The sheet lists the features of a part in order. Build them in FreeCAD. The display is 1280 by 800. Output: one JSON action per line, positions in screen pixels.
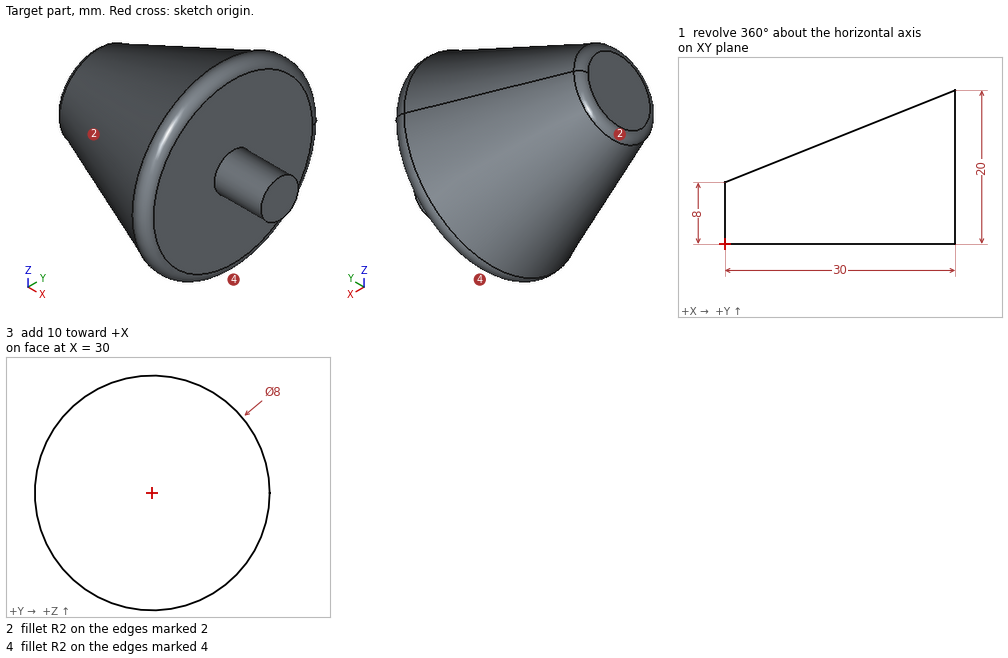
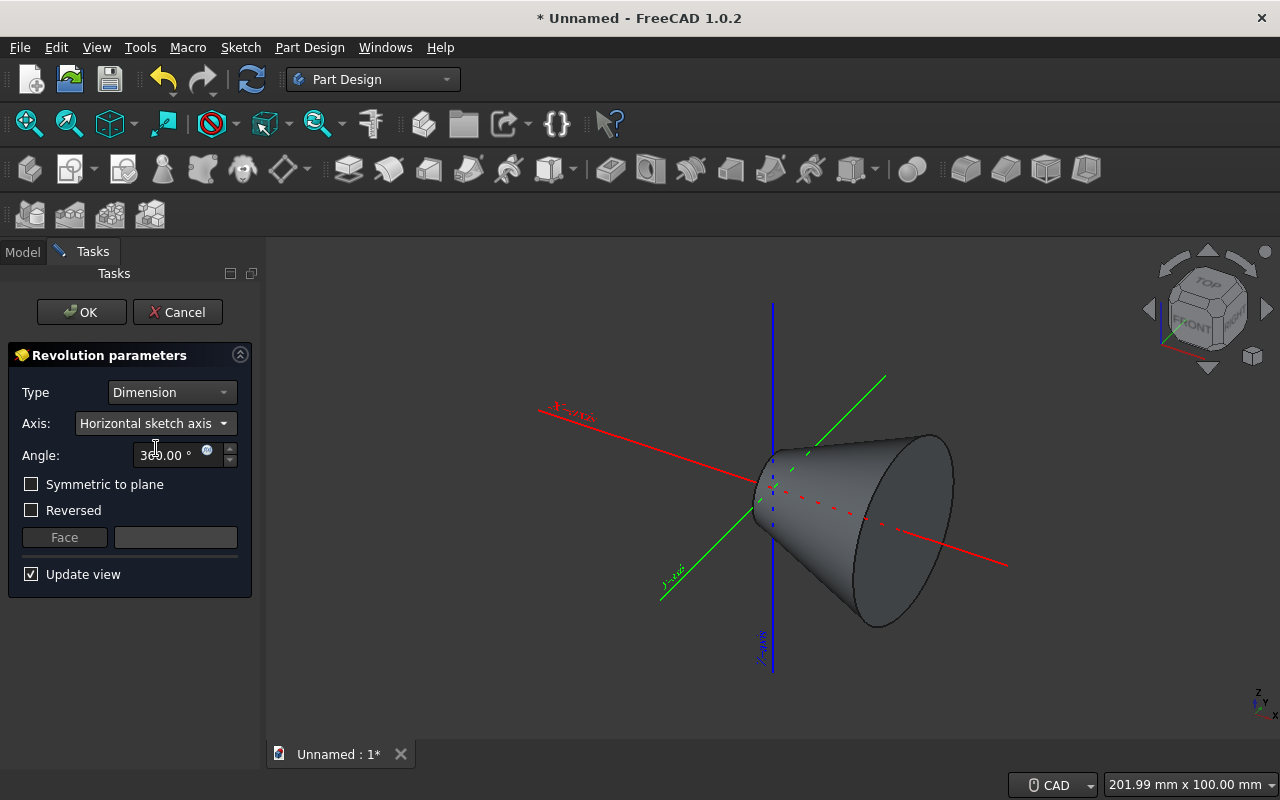
{"action": "left_click", "coordinate": [82, 312]}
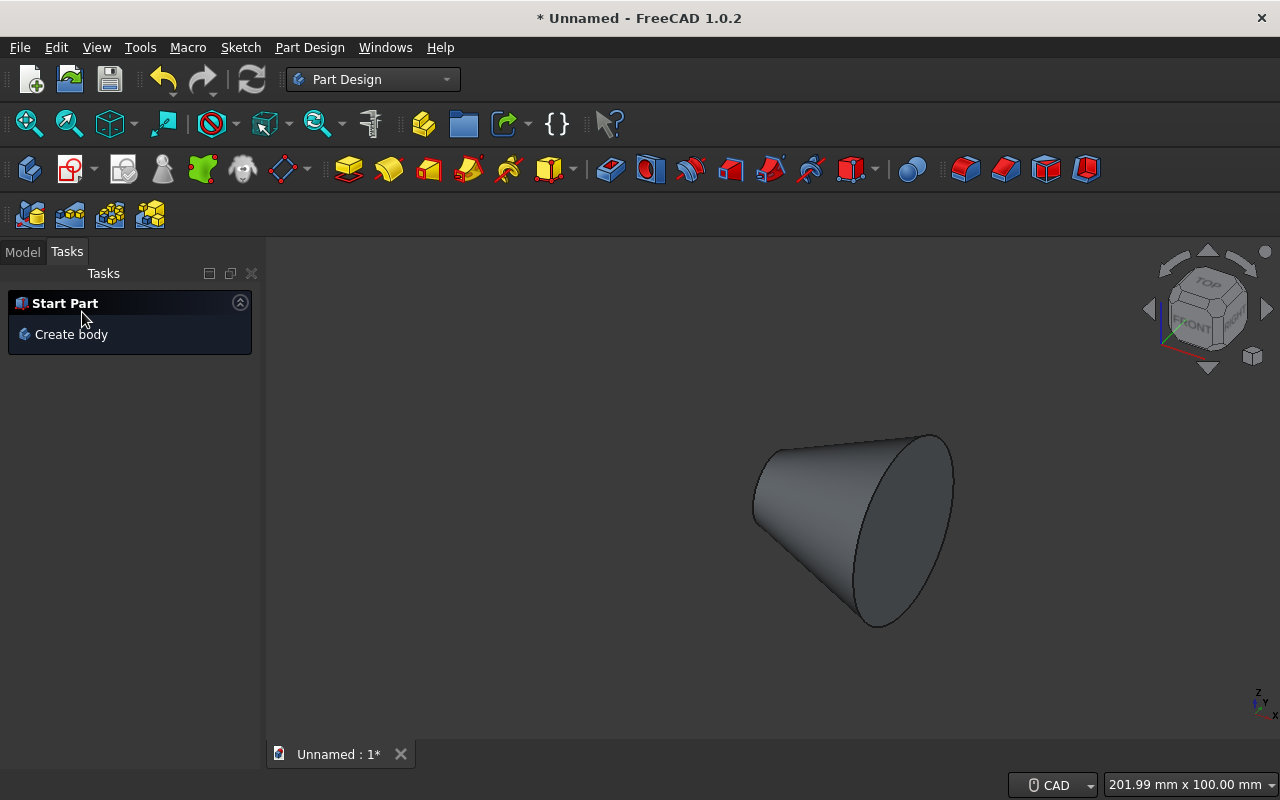
{"action": "left_click", "coordinate": [753, 507]}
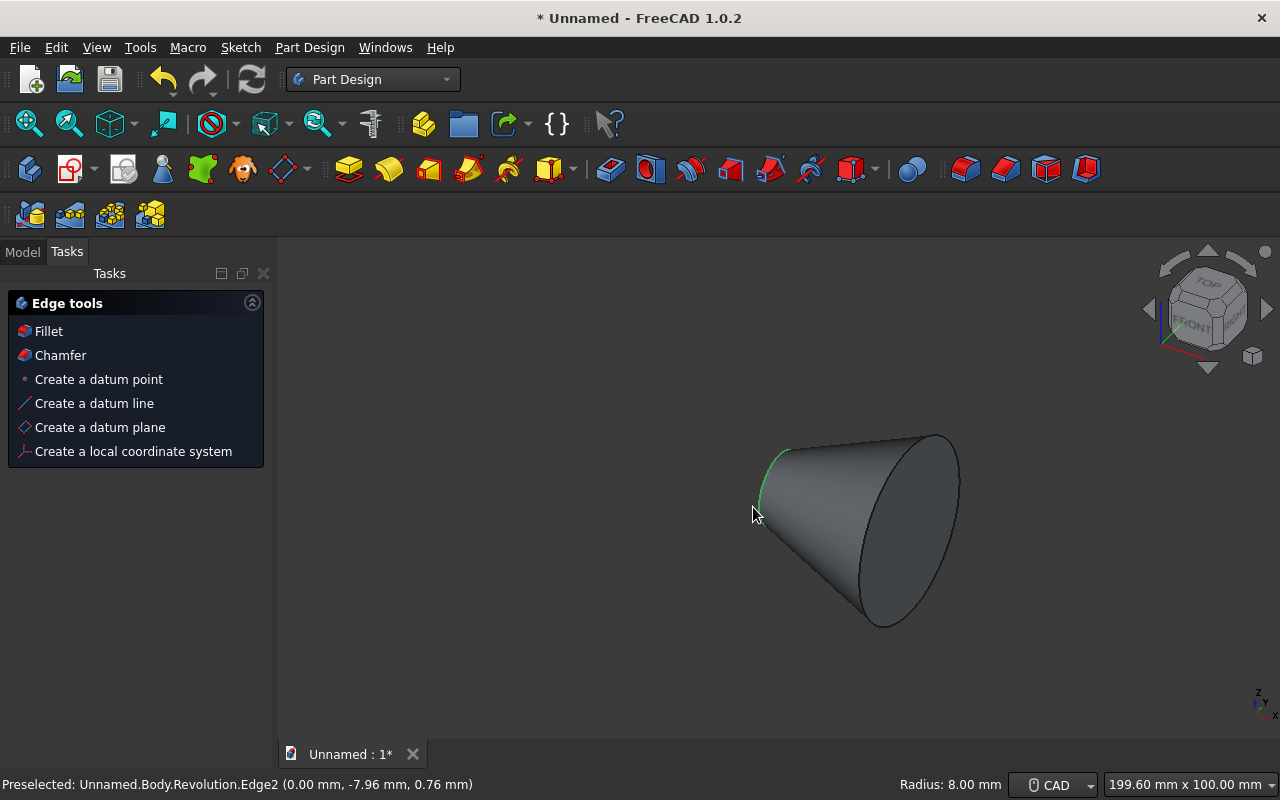
{"action": "left_click", "coordinate": [966, 170]}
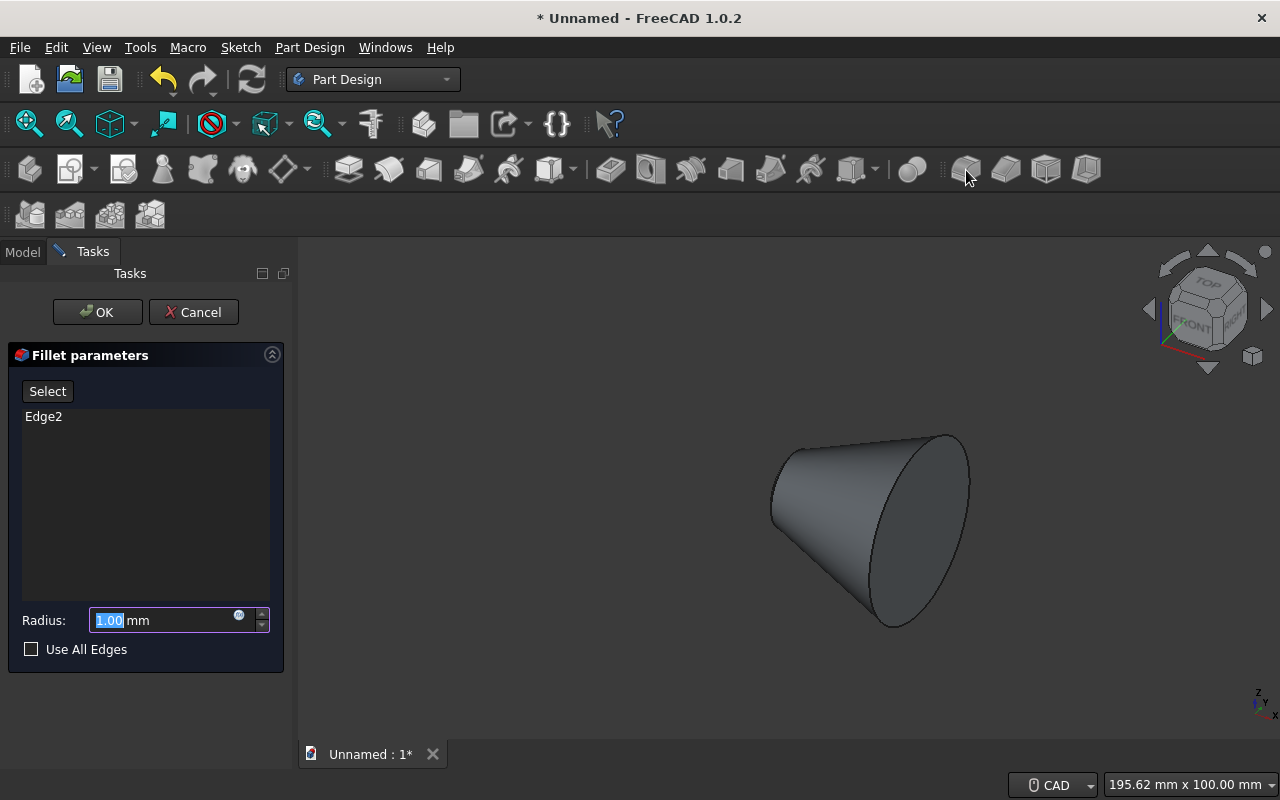
{"action": "type", "text": "2"}
{"action": "key", "text": "Tab"}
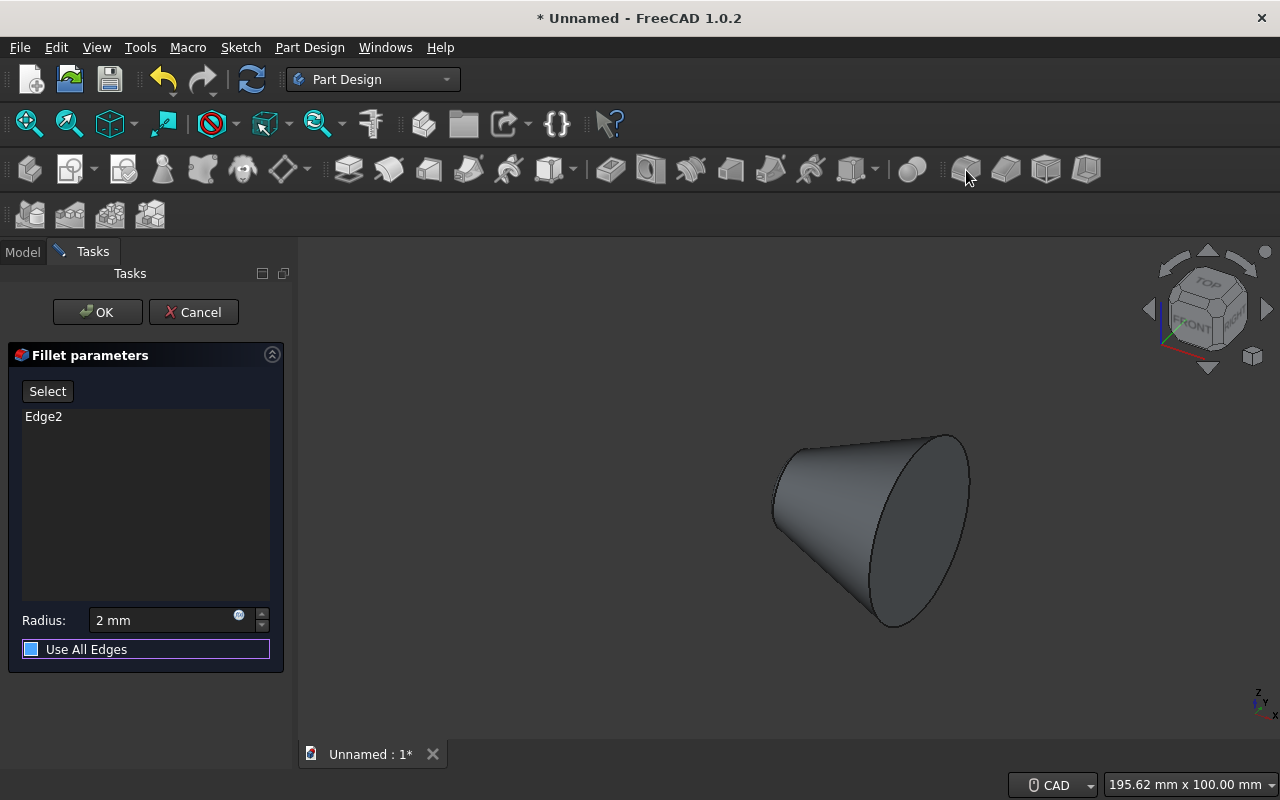
{"action": "left_click", "coordinate": [98, 312]}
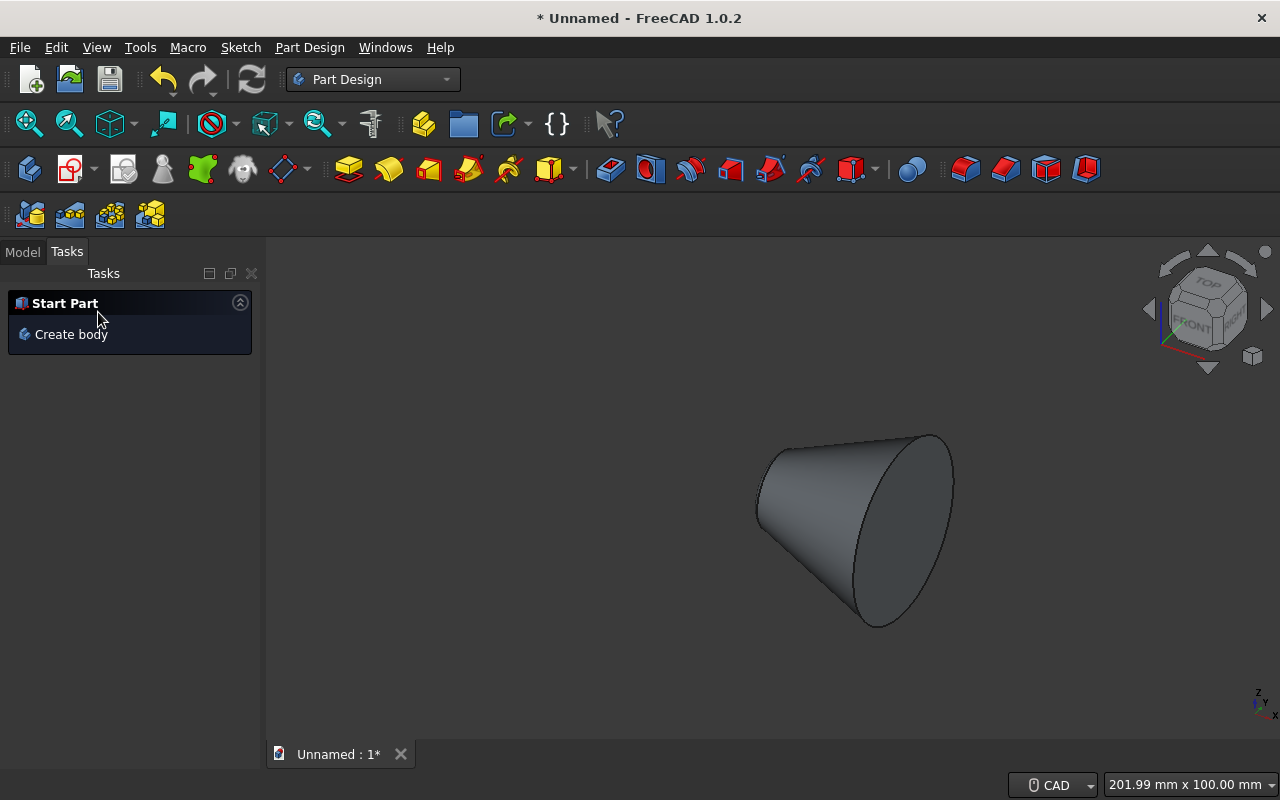
{"action": "left_click", "coordinate": [903, 530]}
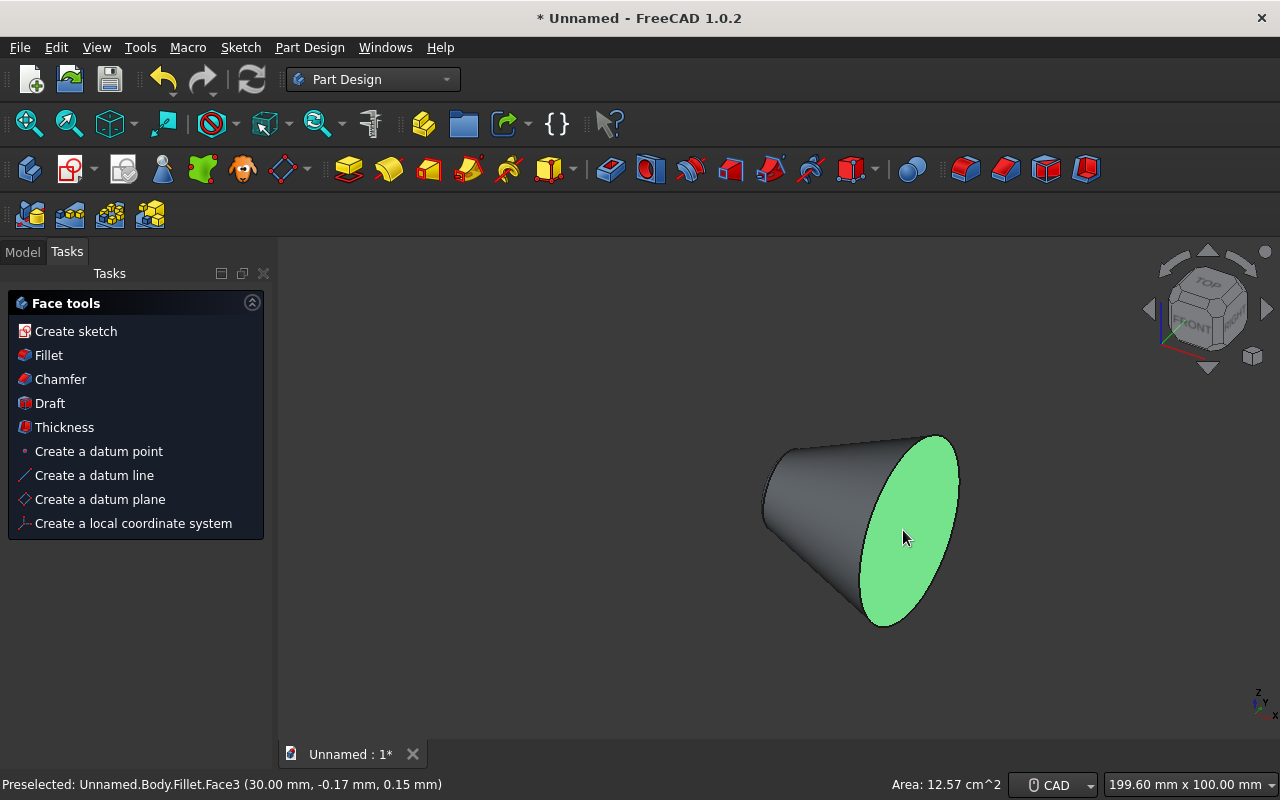
{"action": "left_click", "coordinate": [70, 170]}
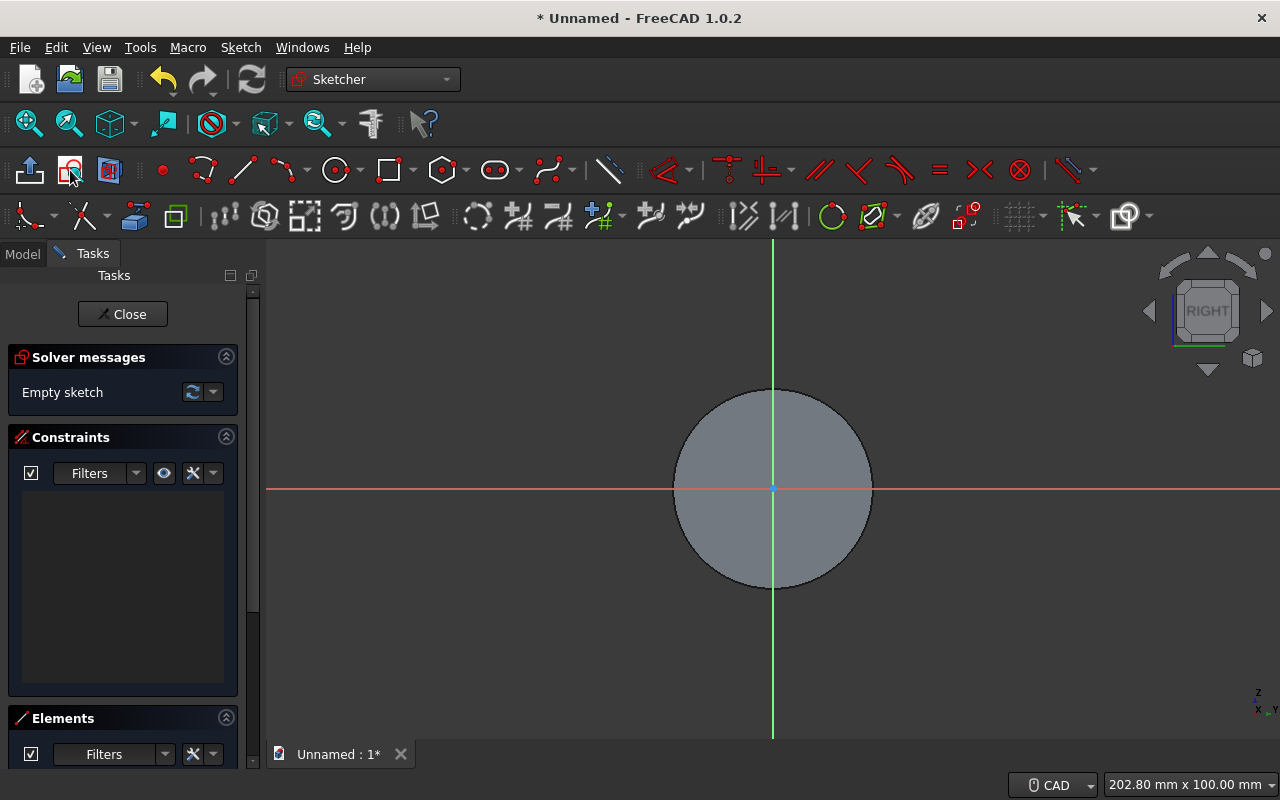
{"action": "scroll", "coordinate": [784, 489], "scroll_direction": "up", "scroll_amount": 10}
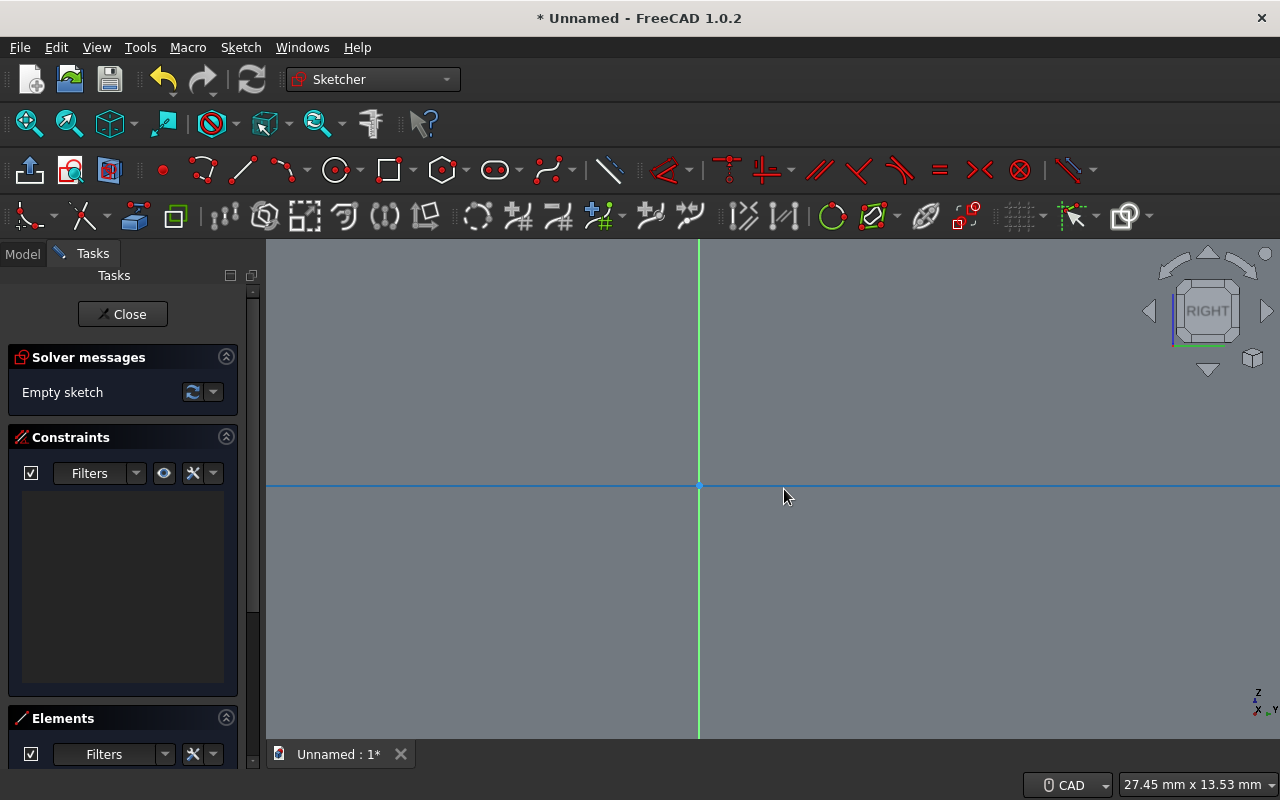
{"action": "left_click", "coordinate": [336, 170]}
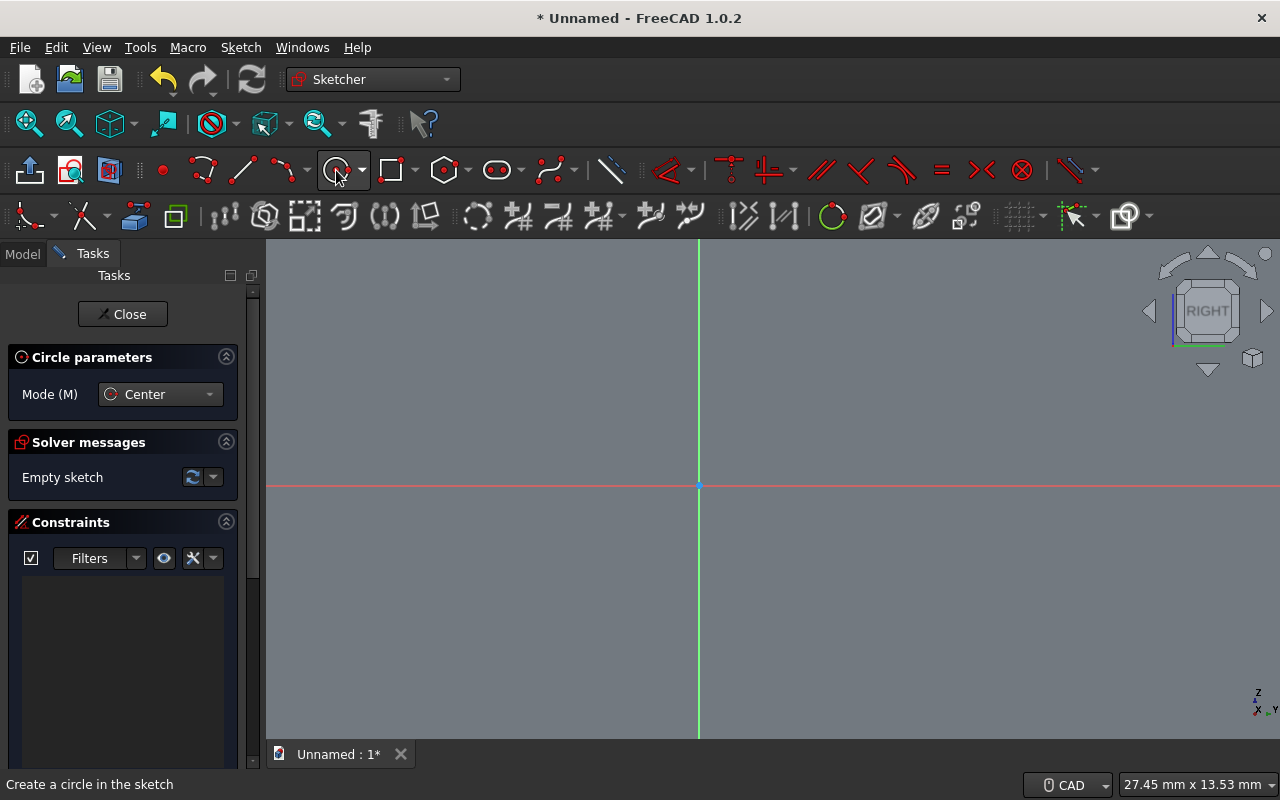
{"action": "left_click", "coordinate": [699, 486]}
{"action": "mouse_move", "coordinate": [804, 381]}